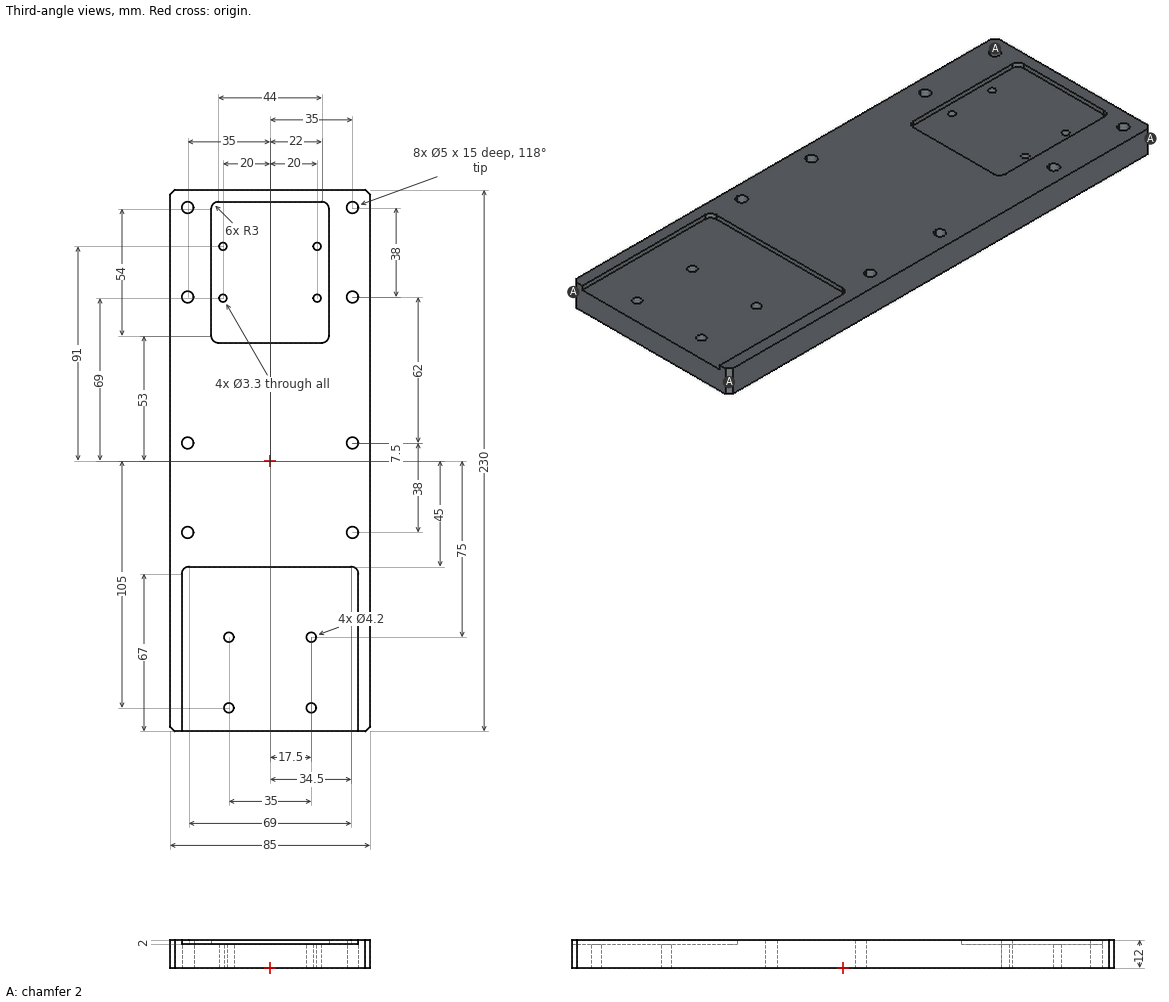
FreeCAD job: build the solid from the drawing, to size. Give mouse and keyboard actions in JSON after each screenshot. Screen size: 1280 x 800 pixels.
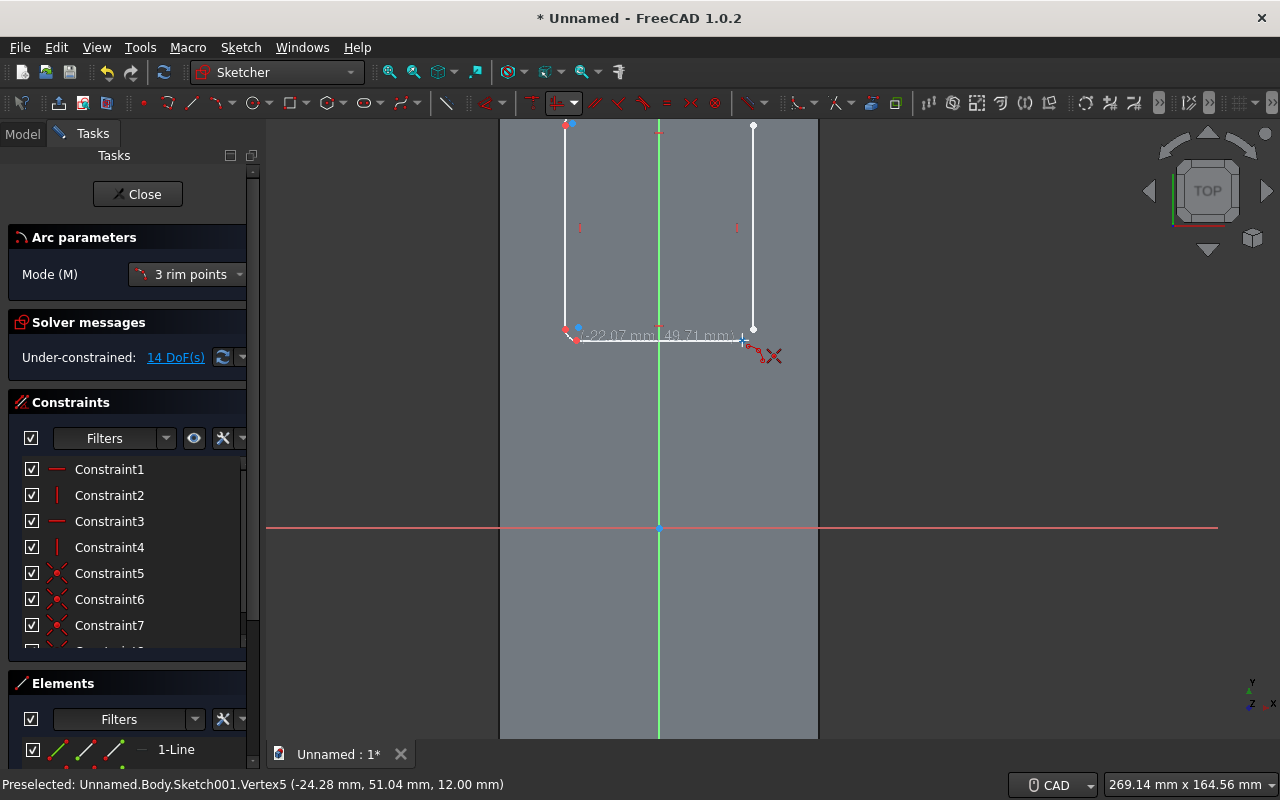
{"action": "left_click", "coordinate": [742, 341]}
{"action": "left_click", "coordinate": [753, 330]}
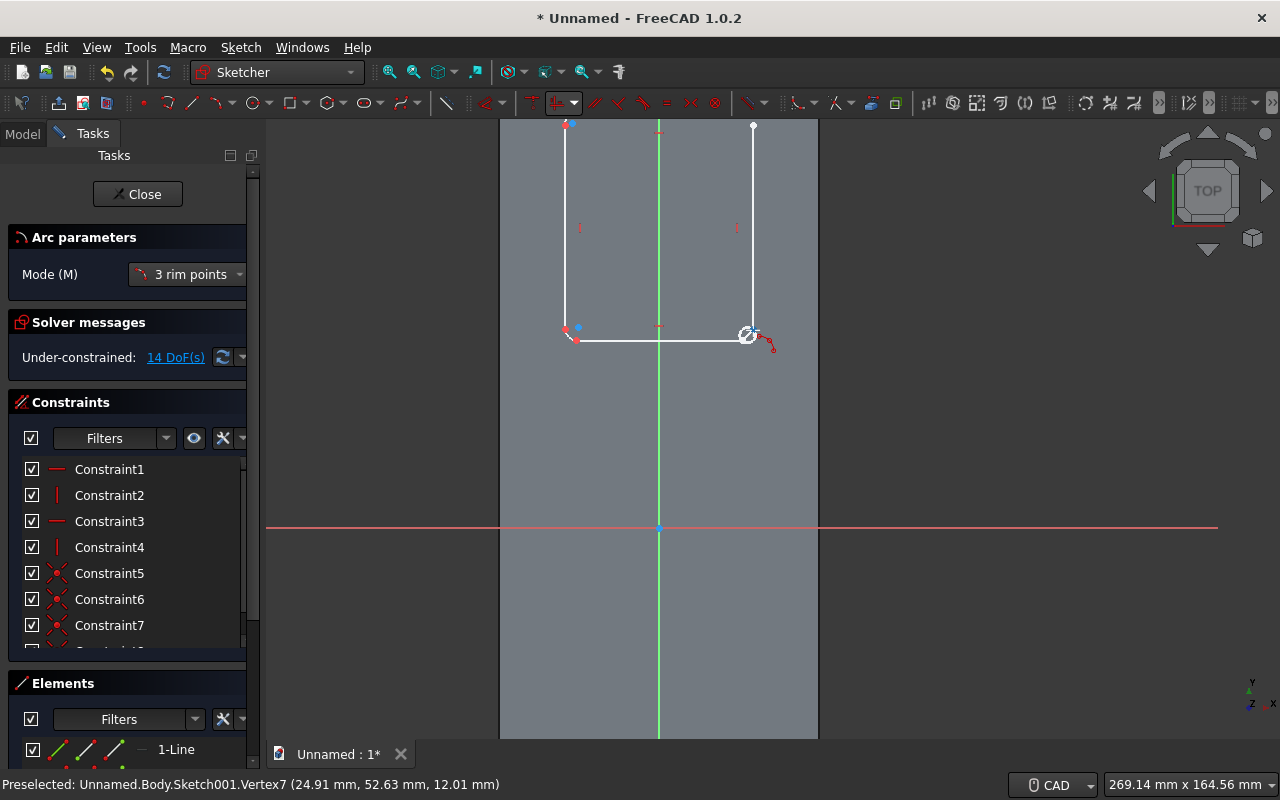
{"action": "scroll", "coordinate": [750, 336], "scroll_direction": "up", "scroll_amount": 8}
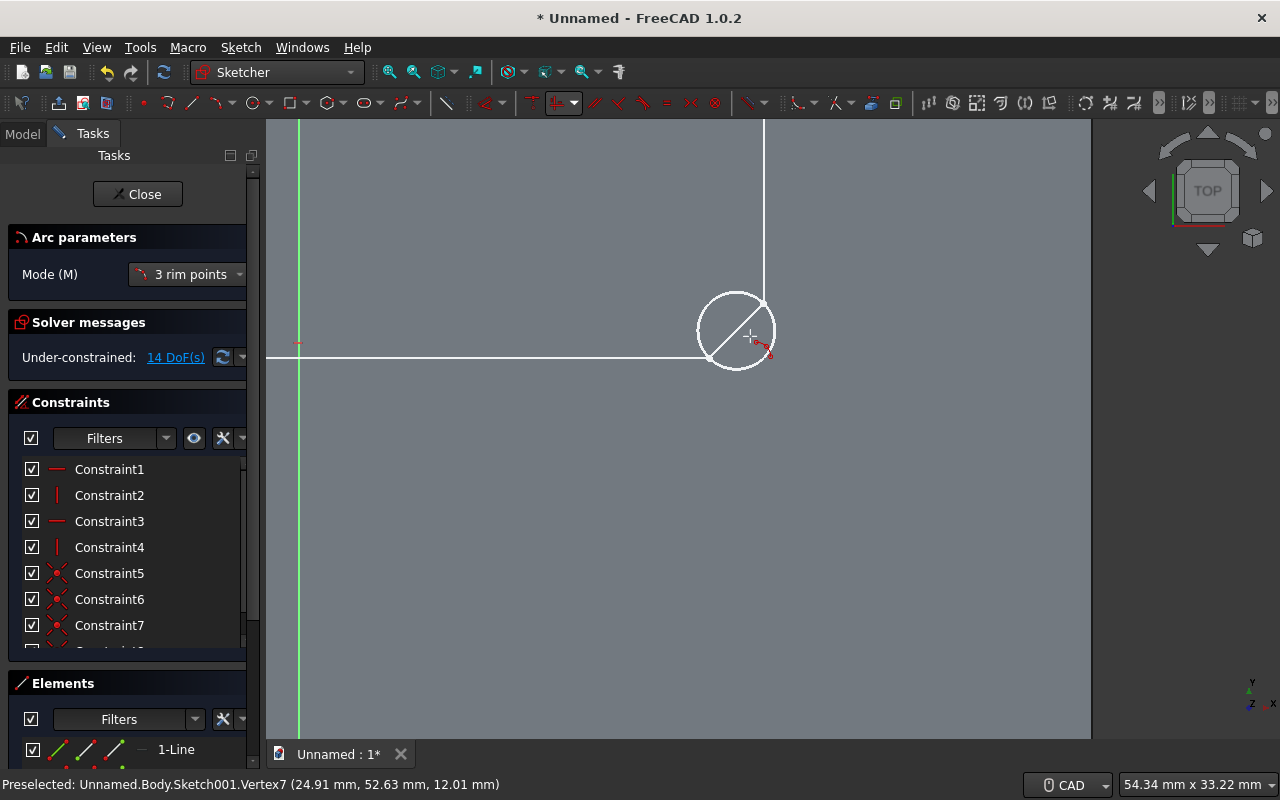
{"action": "left_click", "coordinate": [749, 336]}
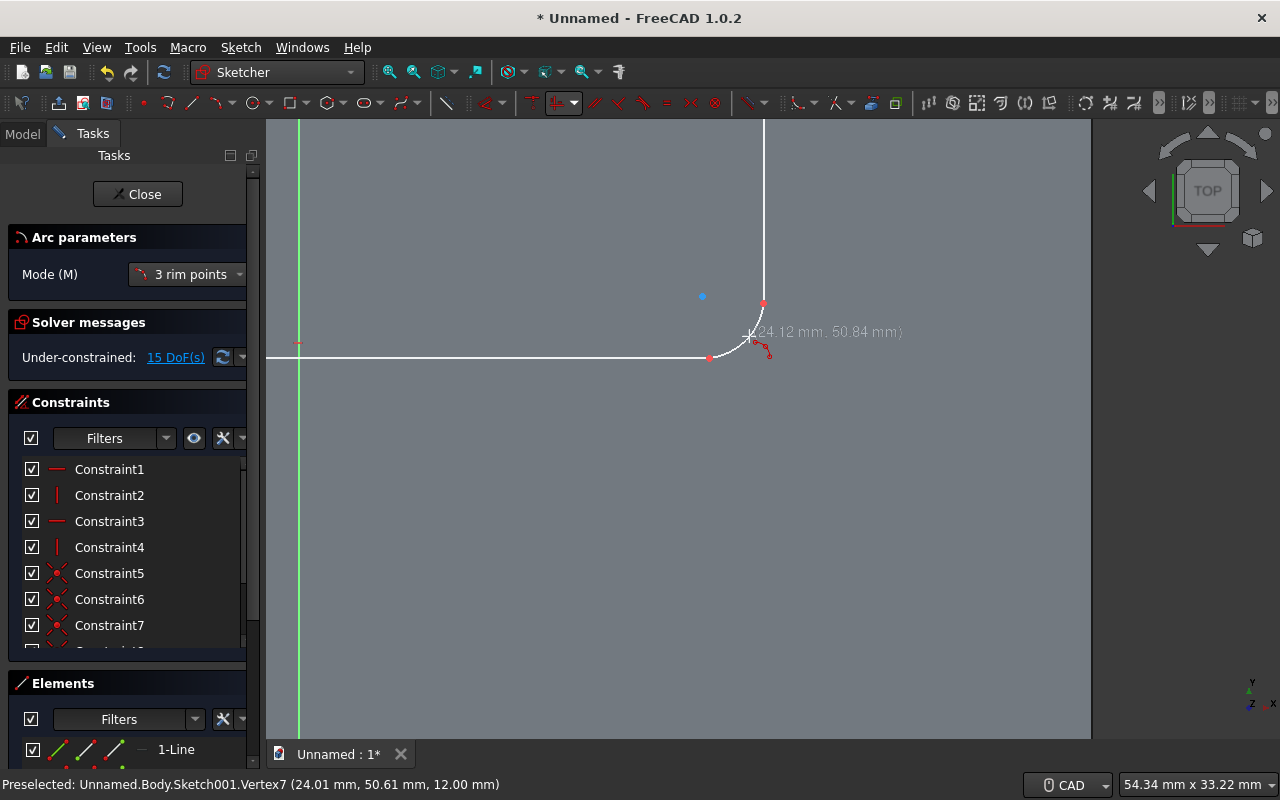
{"action": "scroll", "coordinate": [745, 339], "scroll_direction": "down", "scroll_amount": 12}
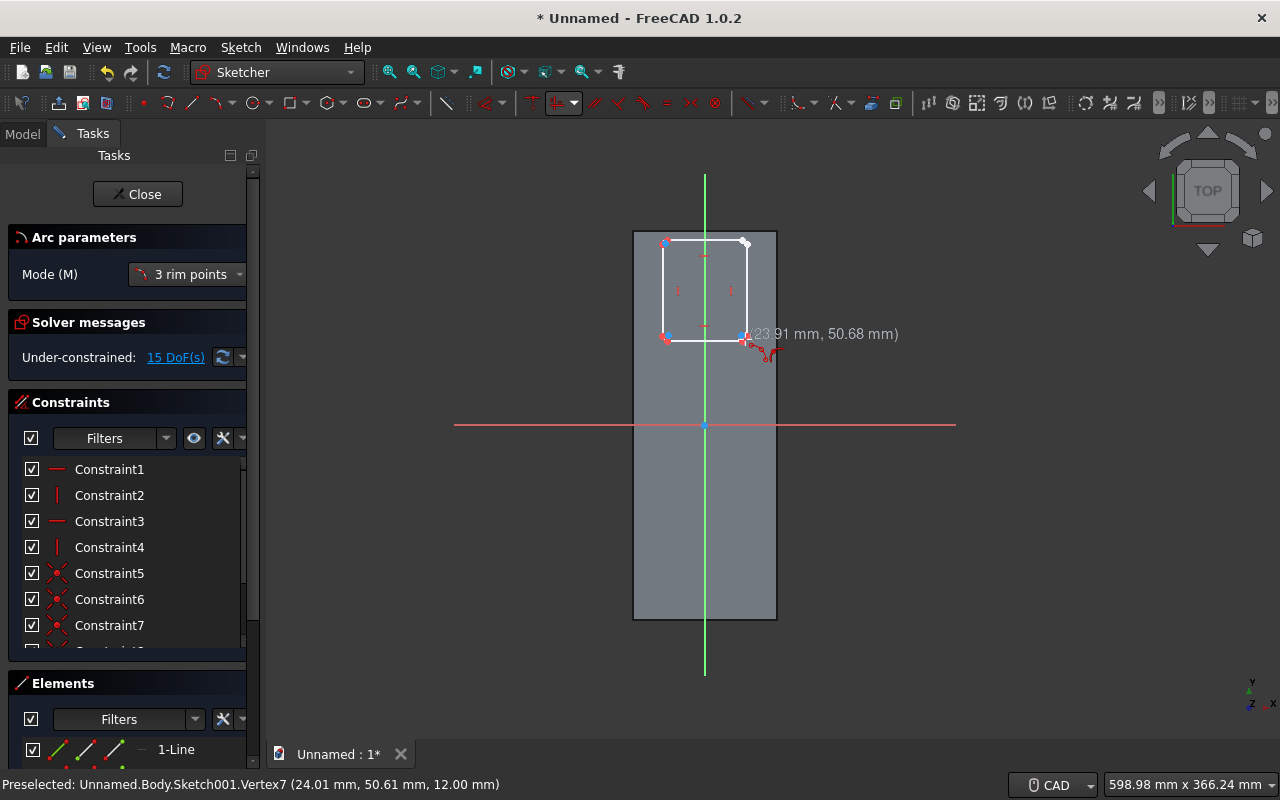
{"action": "scroll", "coordinate": [747, 244], "scroll_direction": "up", "scroll_amount": 4}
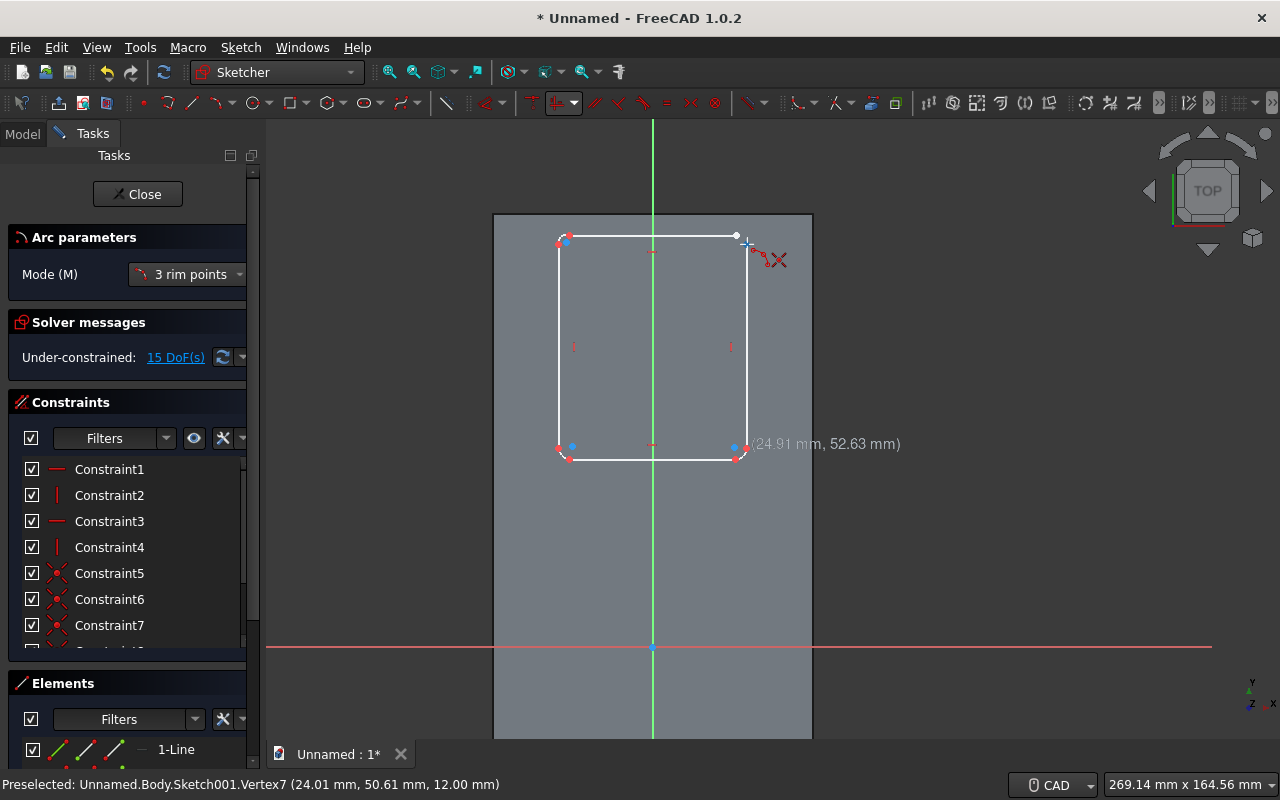
{"action": "left_click", "coordinate": [747, 245]}
{"action": "left_click", "coordinate": [736, 236]}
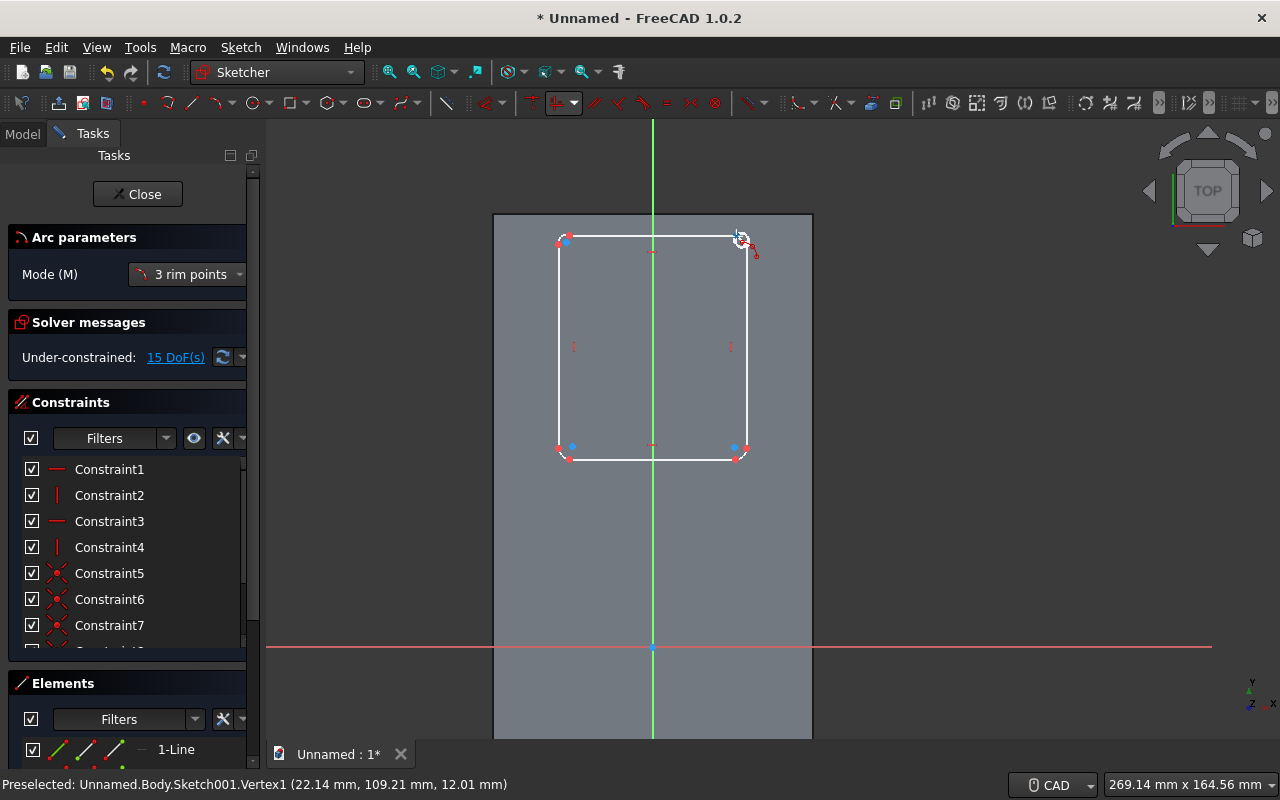
{"action": "scroll", "coordinate": [744, 236], "scroll_direction": "up", "scroll_amount": 8}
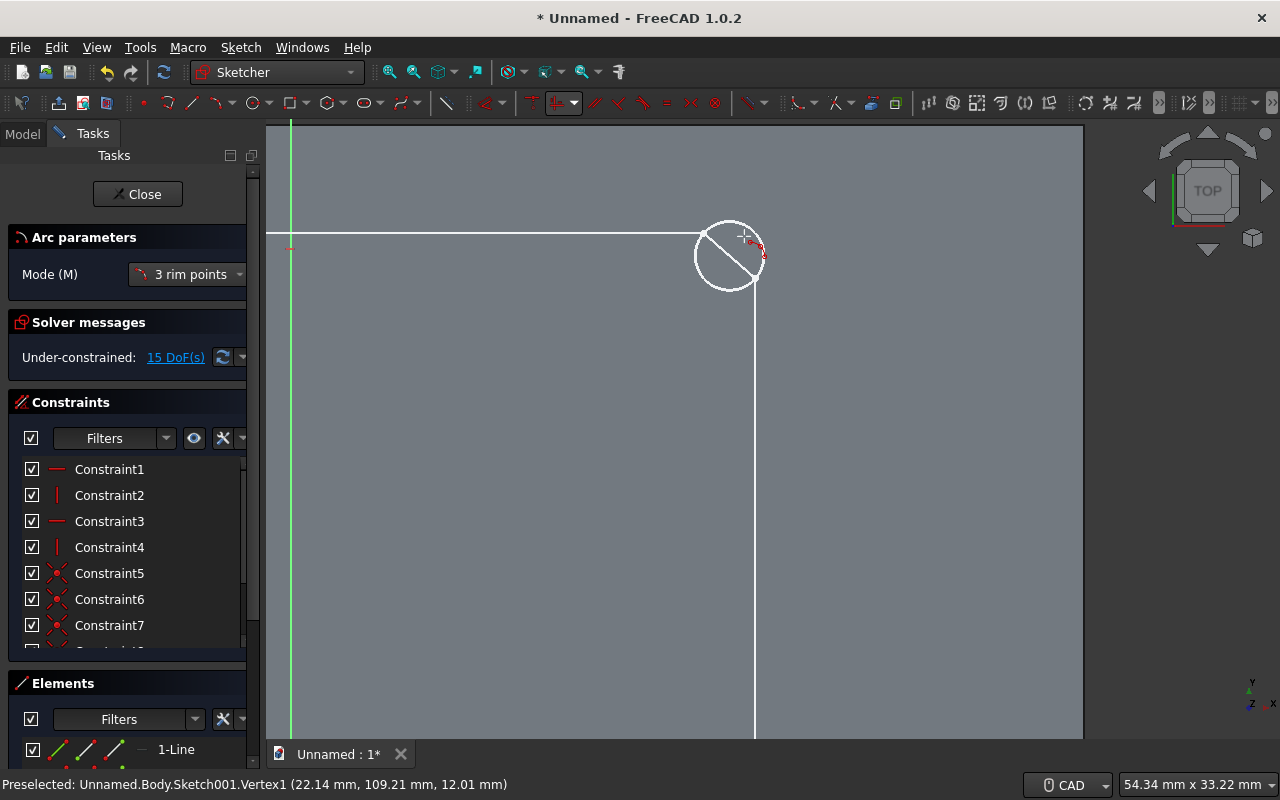
{"action": "left_click", "coordinate": [741, 235]}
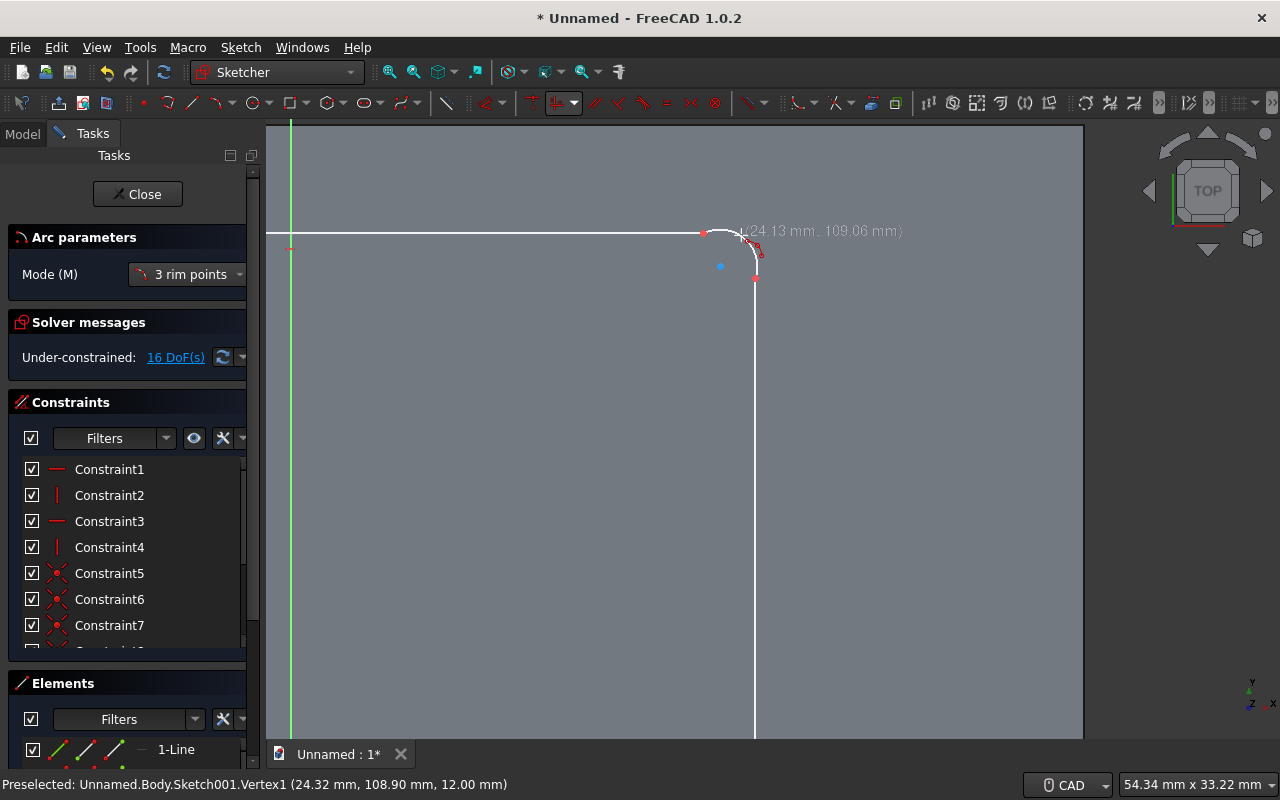
{"action": "key", "text": "g l"}